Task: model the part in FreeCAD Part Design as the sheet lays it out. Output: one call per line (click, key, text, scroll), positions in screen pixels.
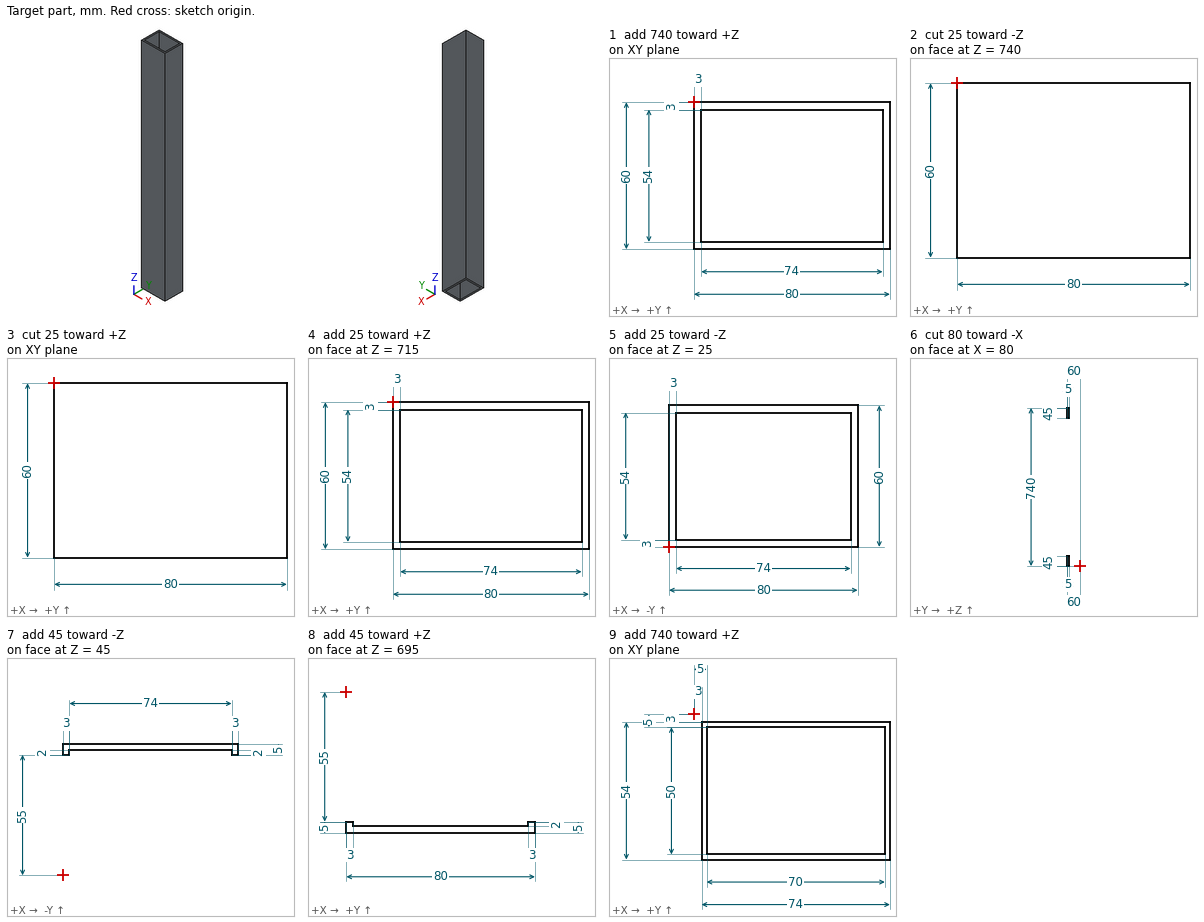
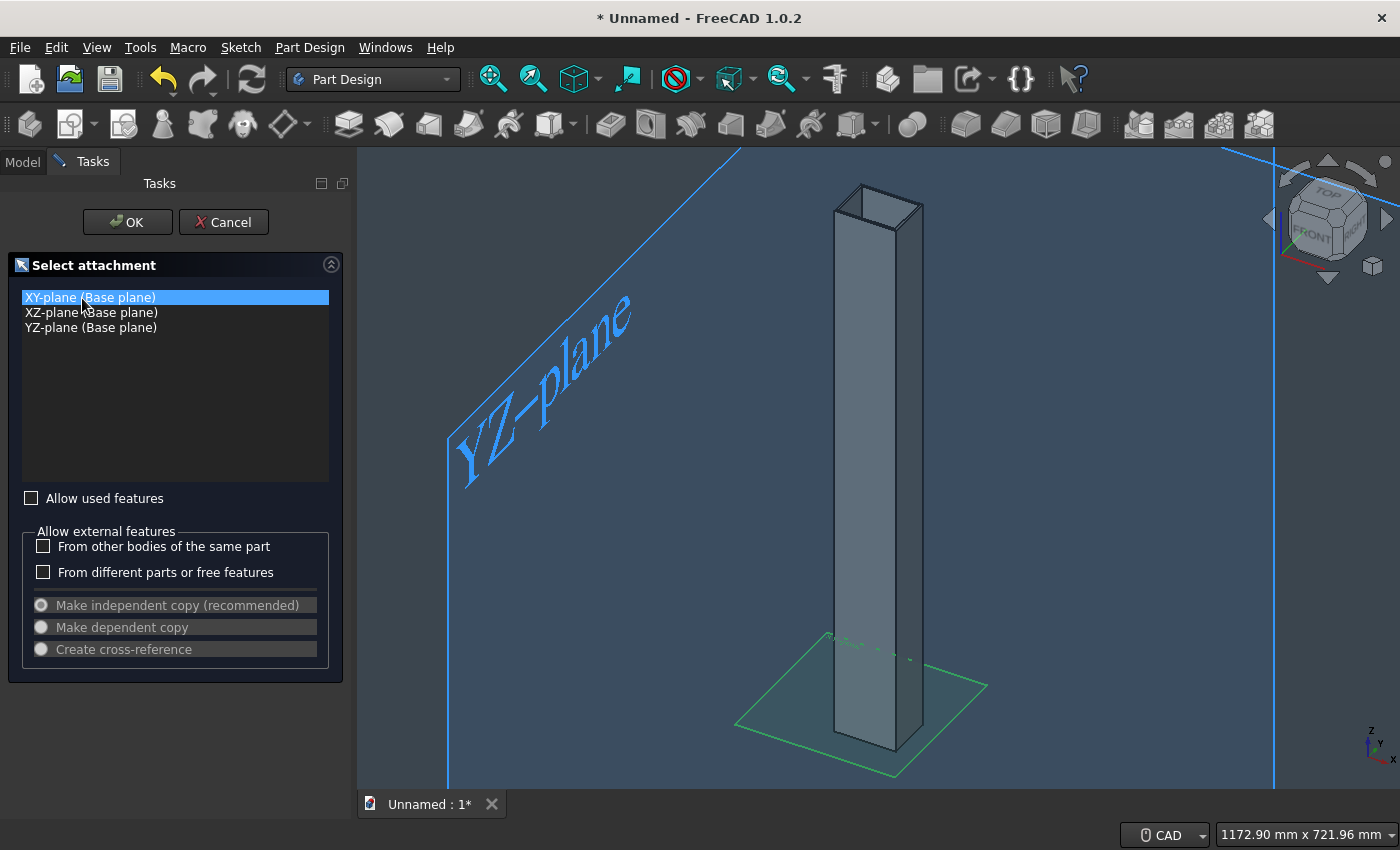
click(128, 222)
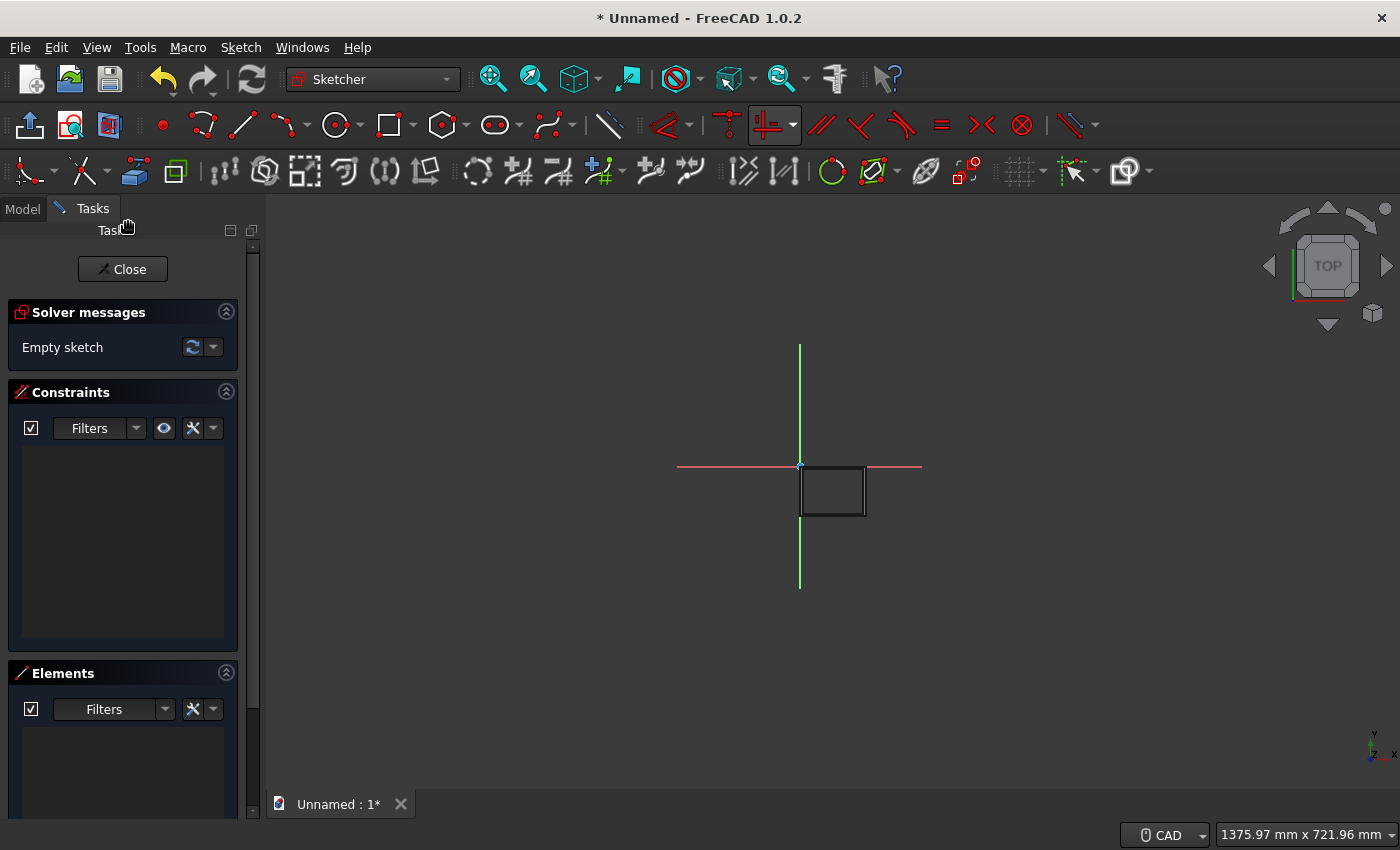
key(q)
key(s)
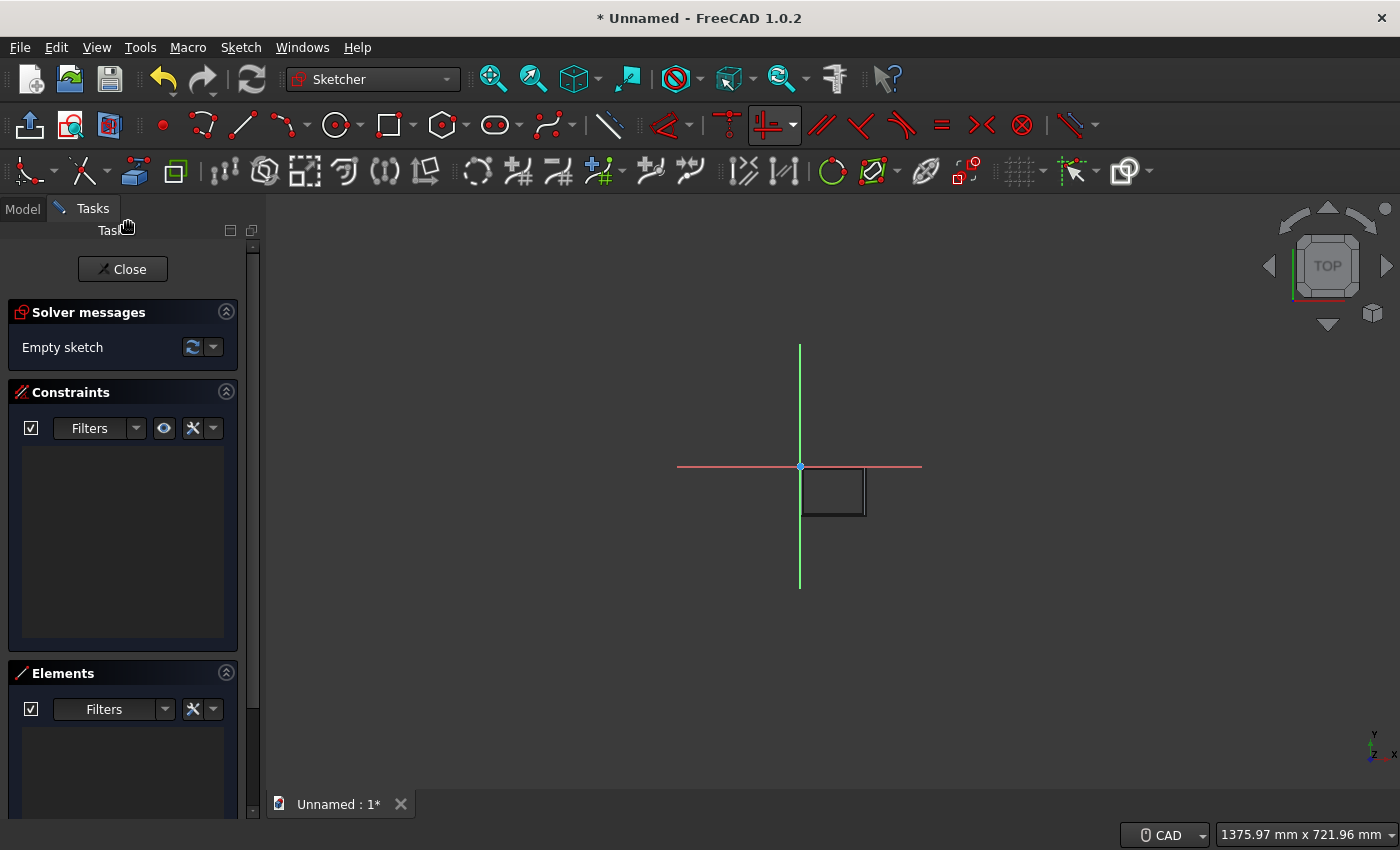
scroll(844, 492, up, 10)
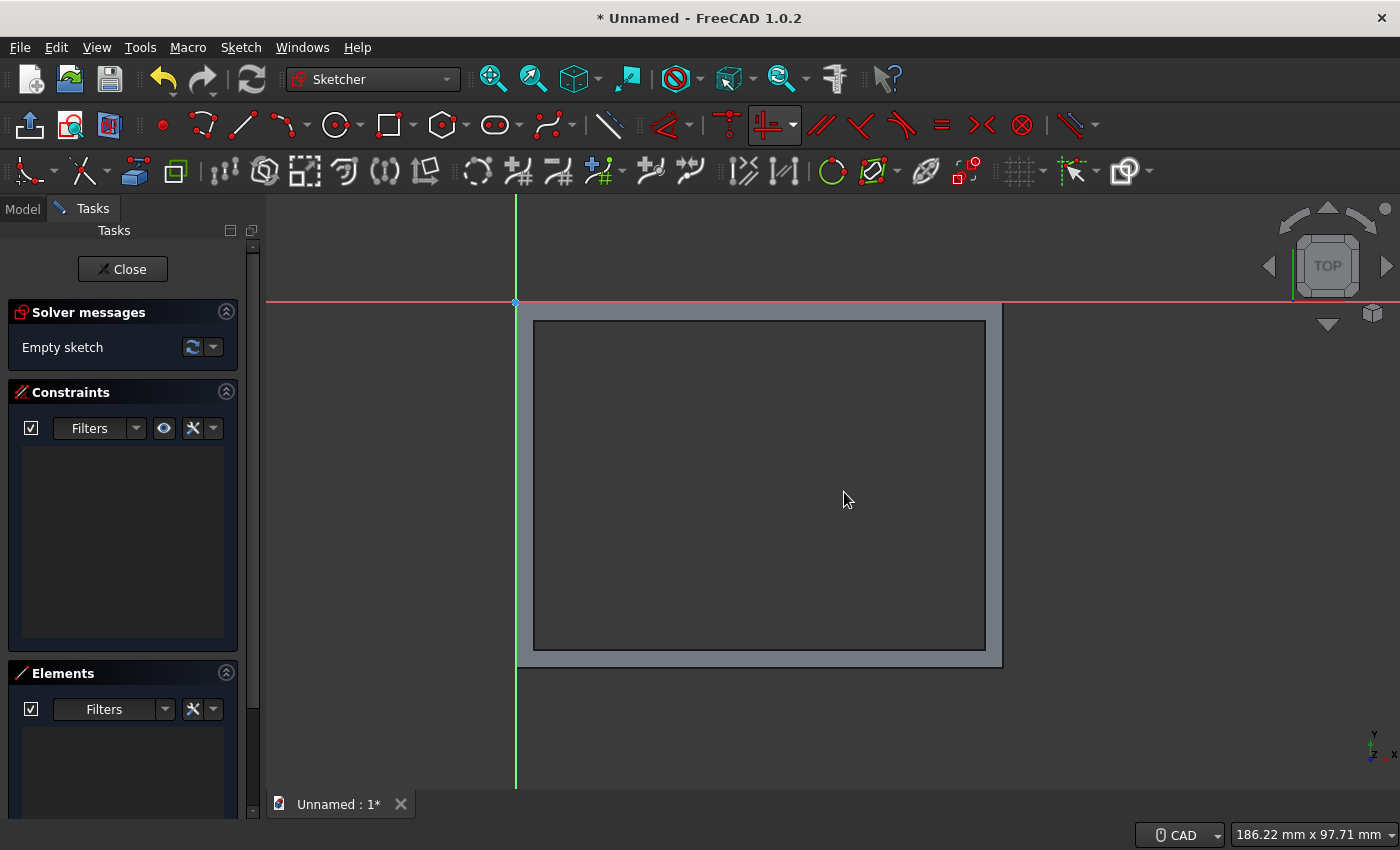
key(g)
key(r)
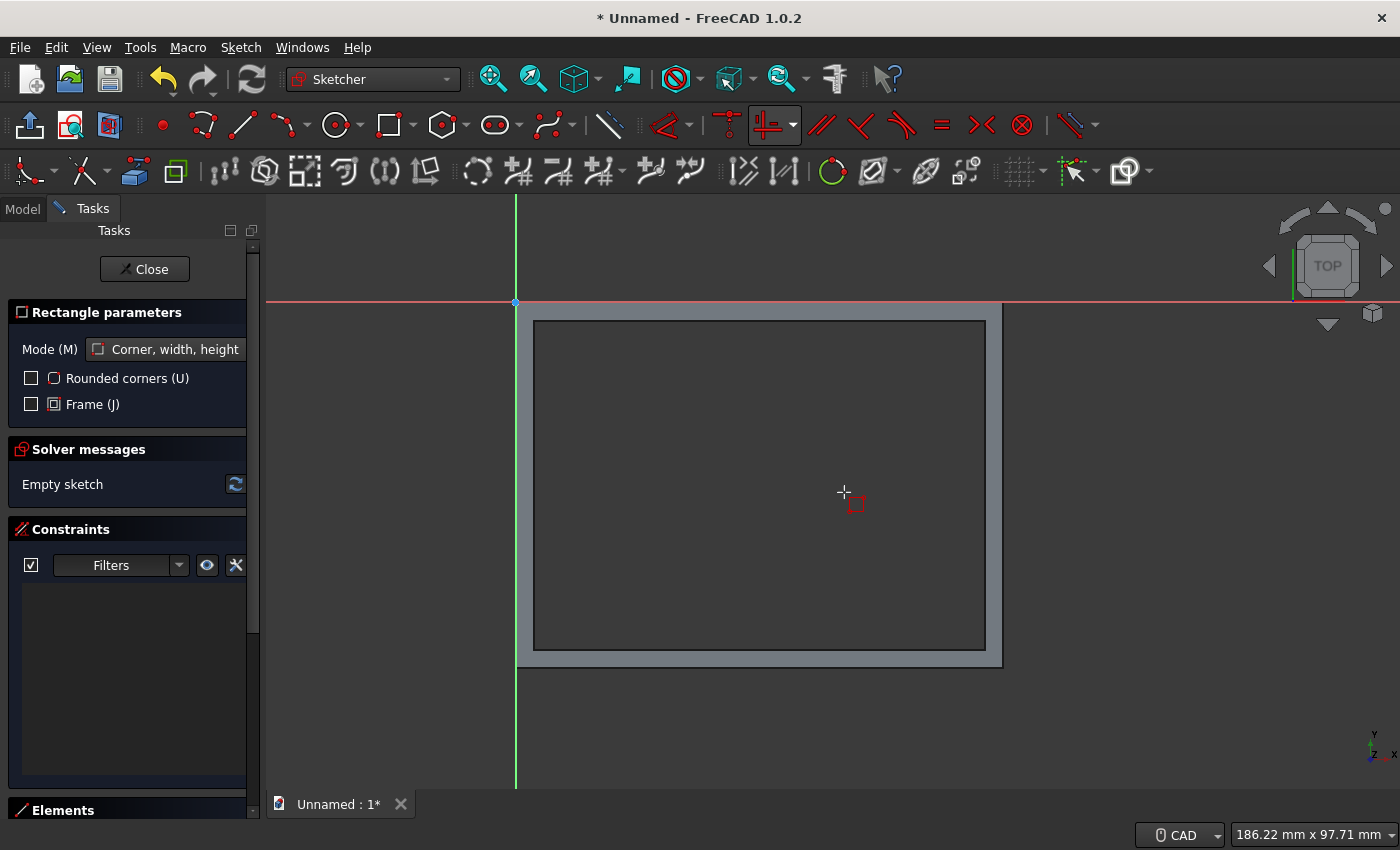
click(516, 302)
click(1003, 668)
key(Escape)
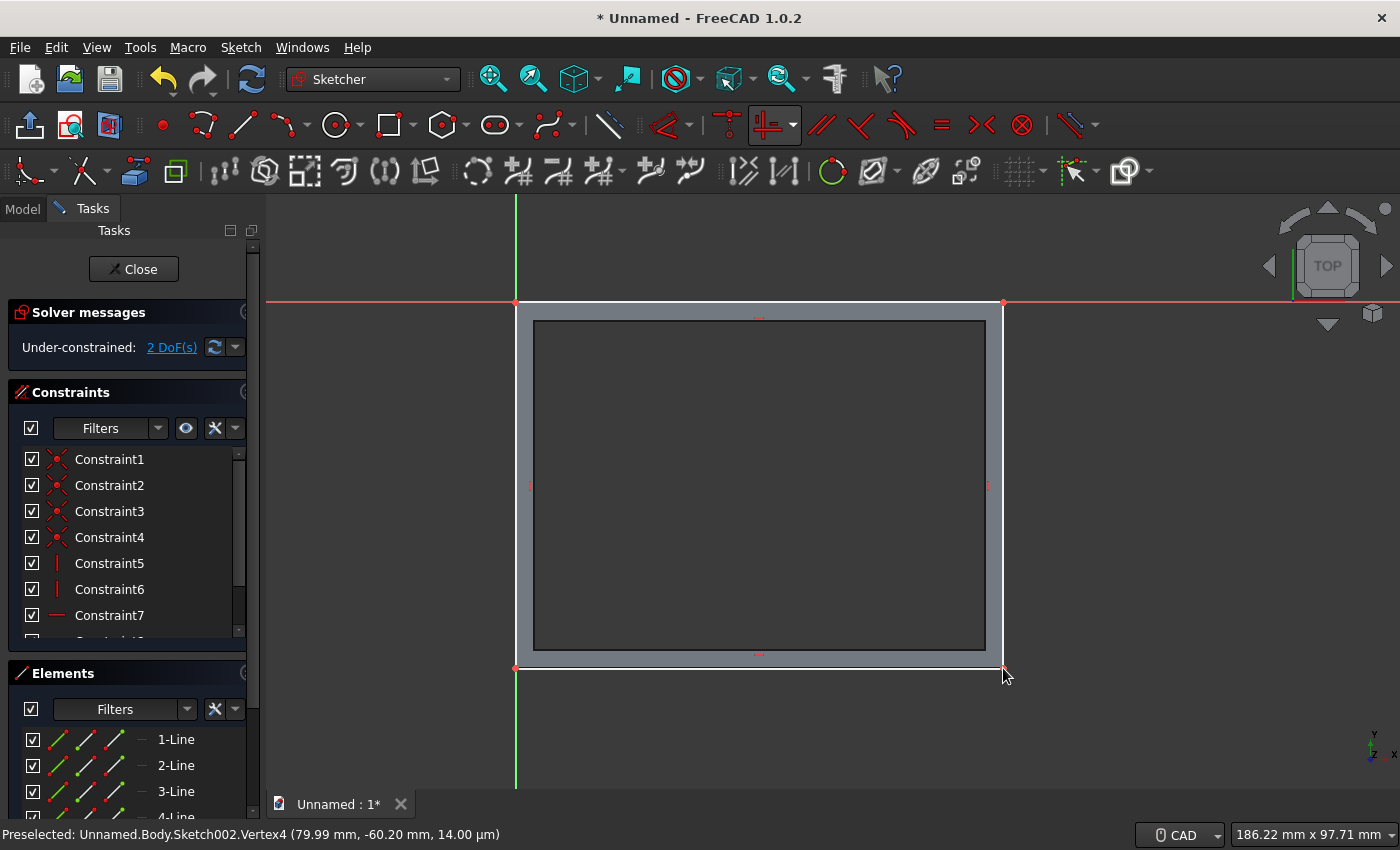
click(664, 126)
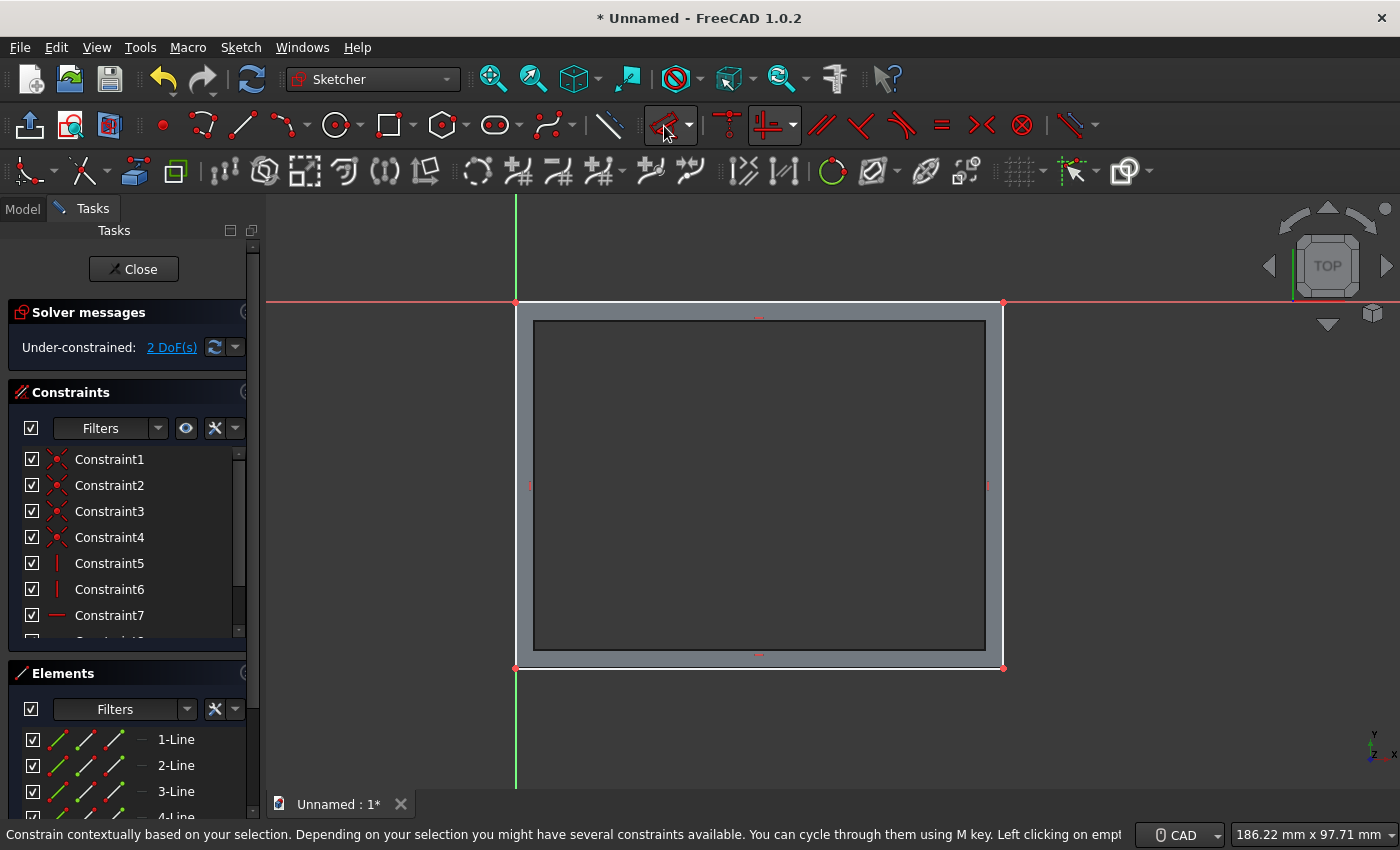
click(516, 412)
click(482, 486)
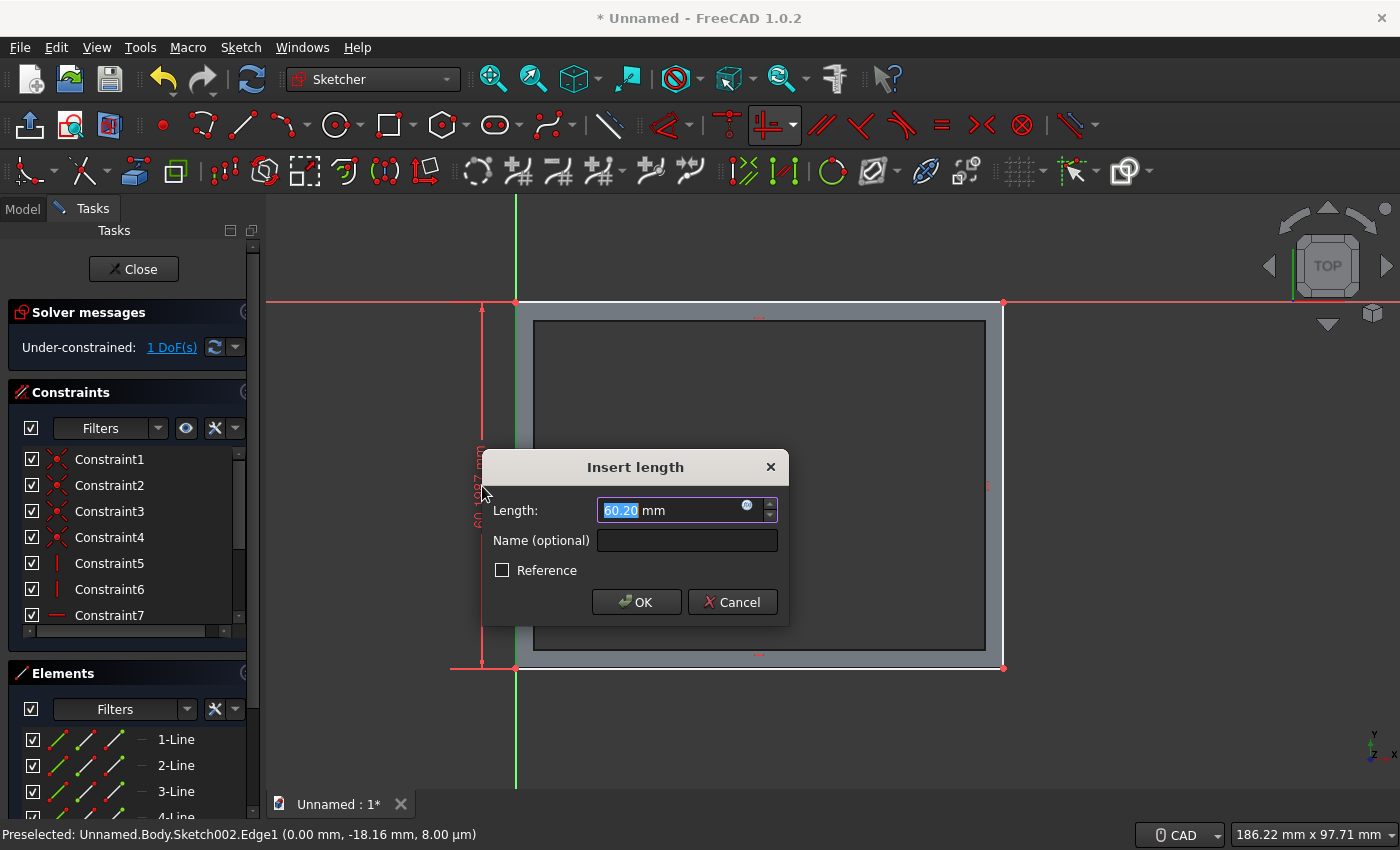
text(60)
key(Return)